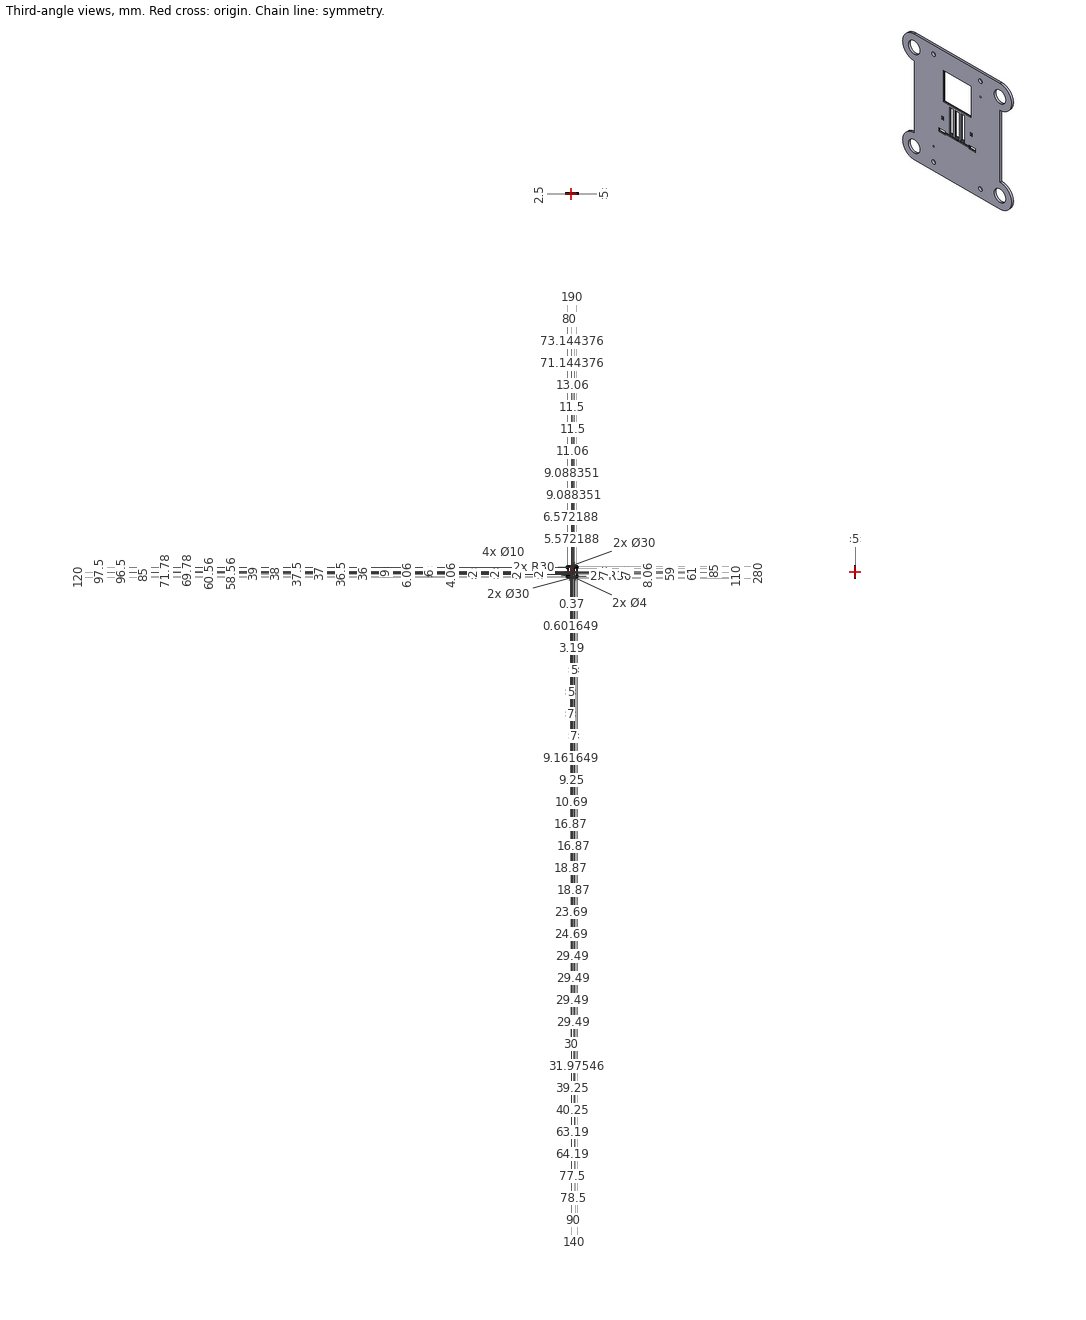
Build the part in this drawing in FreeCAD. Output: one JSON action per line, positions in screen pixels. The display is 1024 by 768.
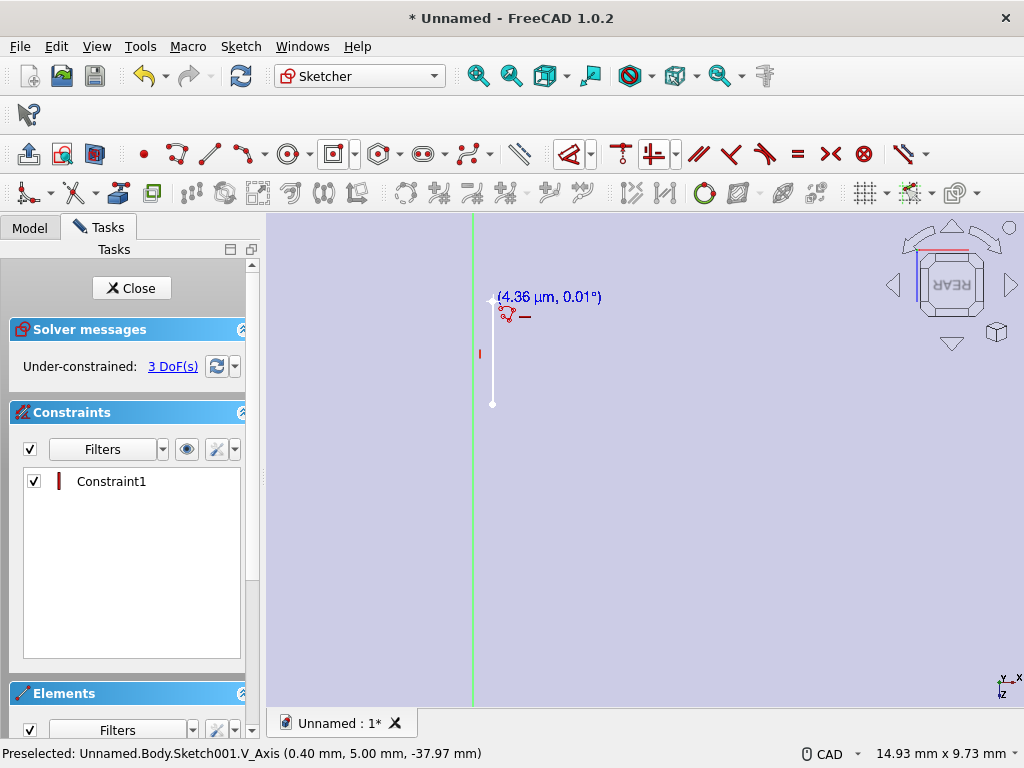
{"action": "scroll", "coordinate": [502, 299], "scroll_direction": "down", "scroll_amount": 15}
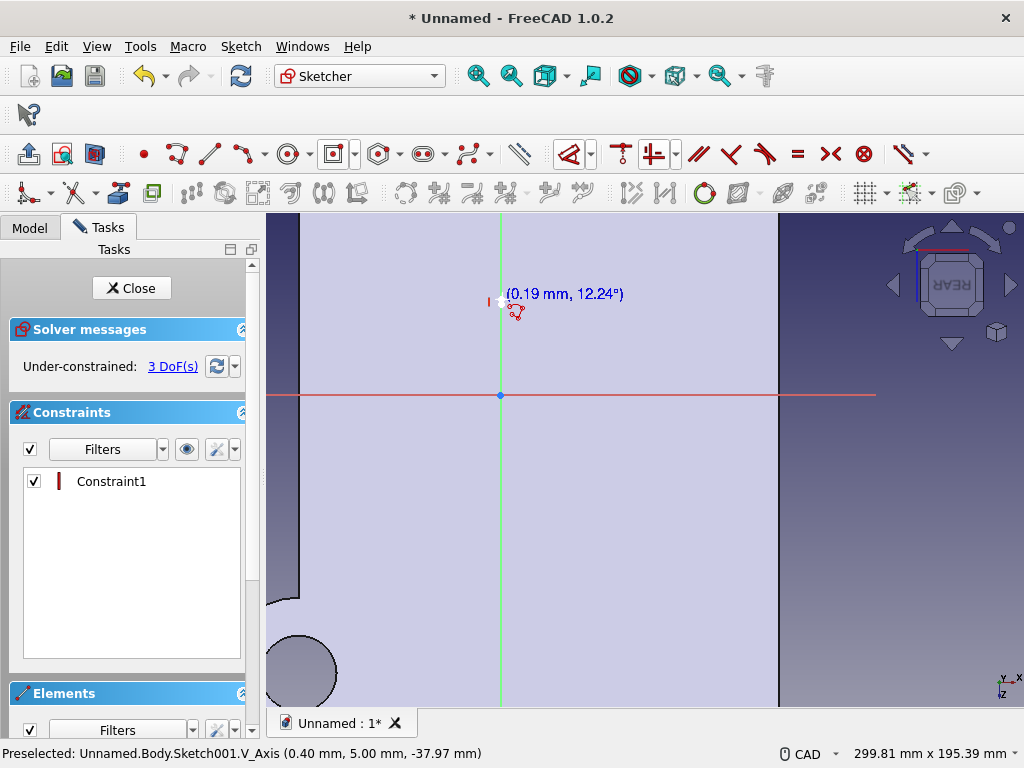
{"action": "left_click", "coordinate": [576, 299]}
{"action": "left_click", "coordinate": [576, 284]}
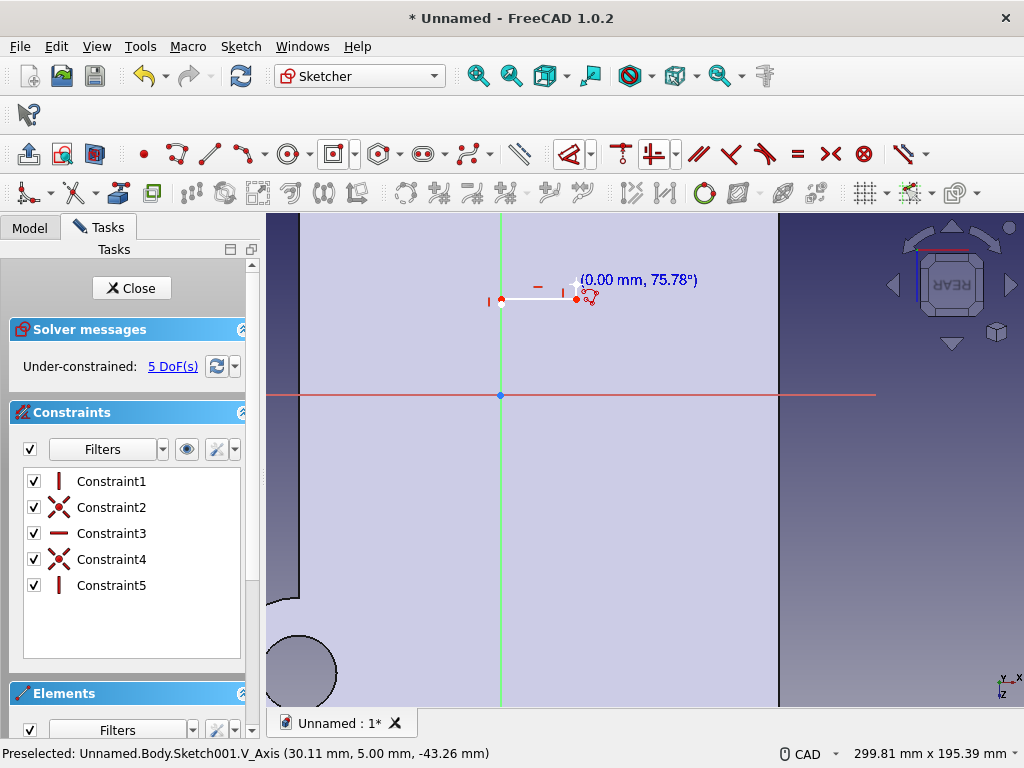
{"action": "scroll", "coordinate": [502, 284], "scroll_direction": "up", "scroll_amount": 15}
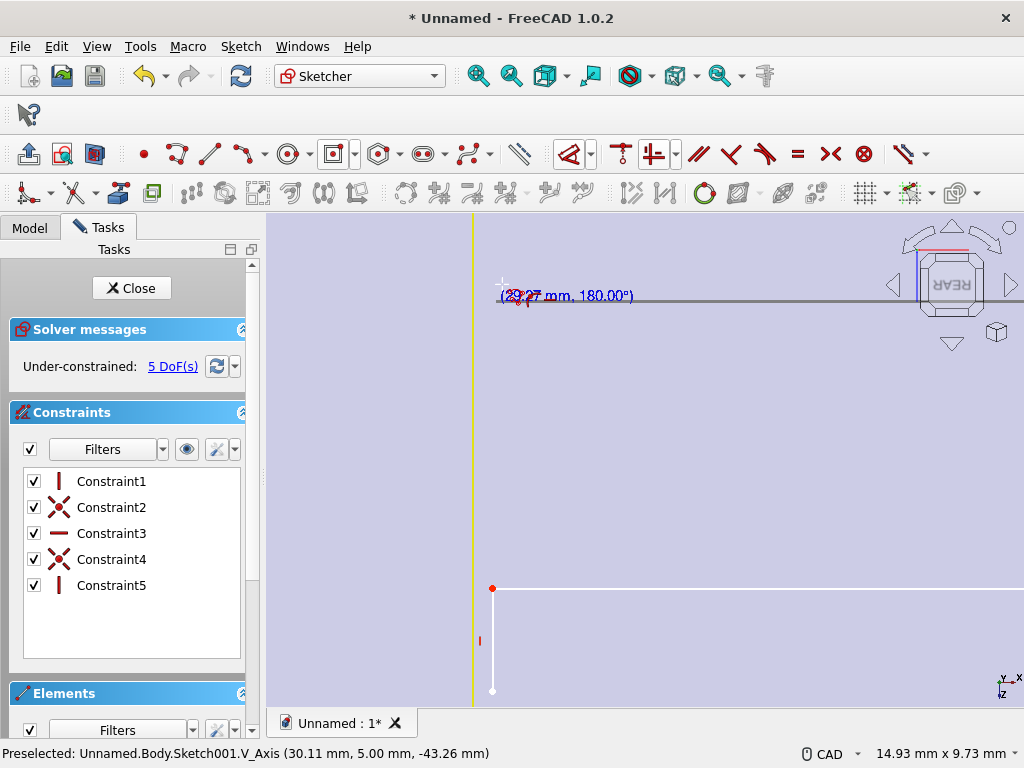
{"action": "left_click", "coordinate": [492, 281]}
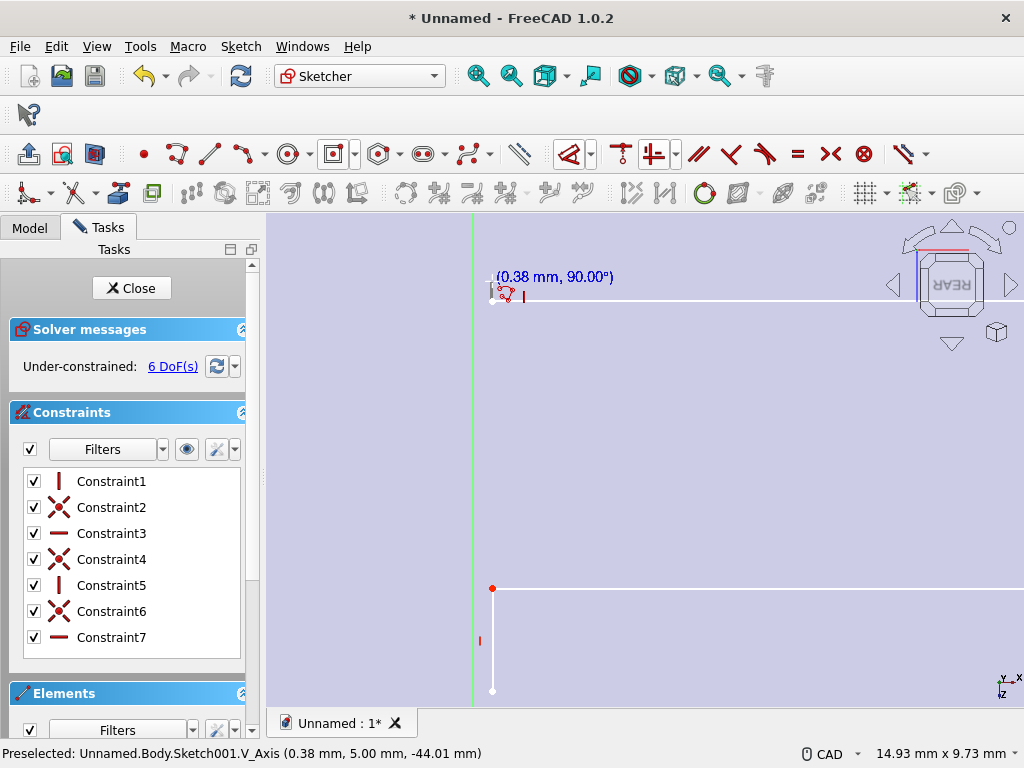
{"action": "scroll", "coordinate": [502, 284], "scroll_direction": "down", "scroll_amount": 15}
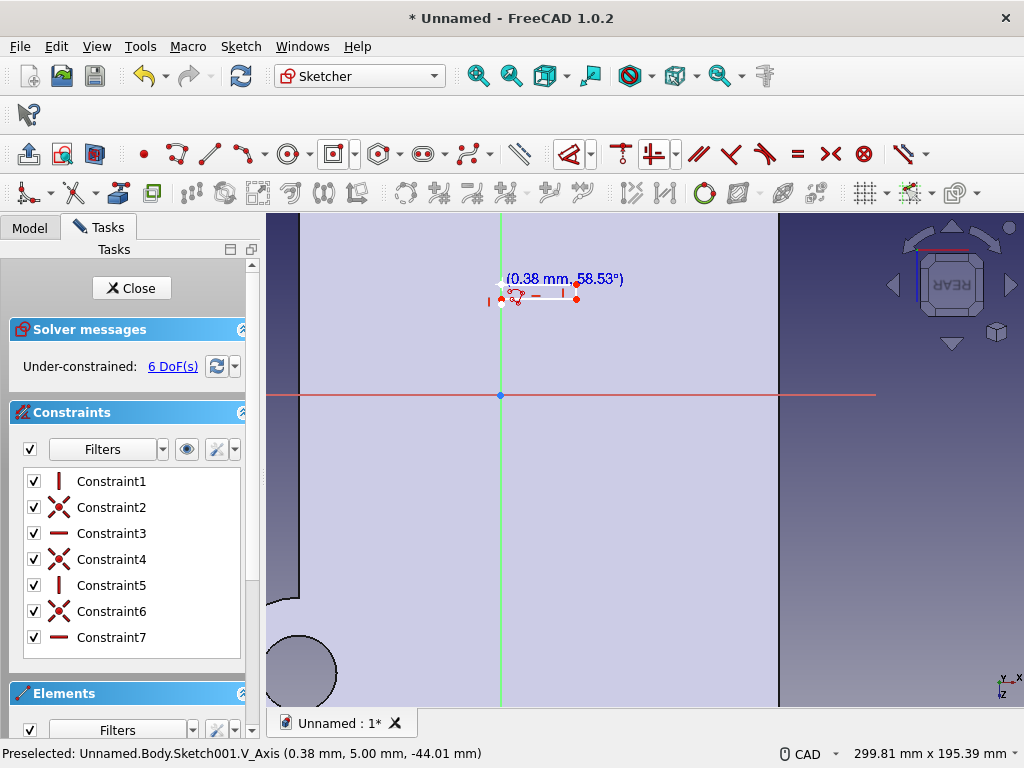
{"action": "scroll", "coordinate": [502, 279], "scroll_direction": "up", "scroll_amount": 15}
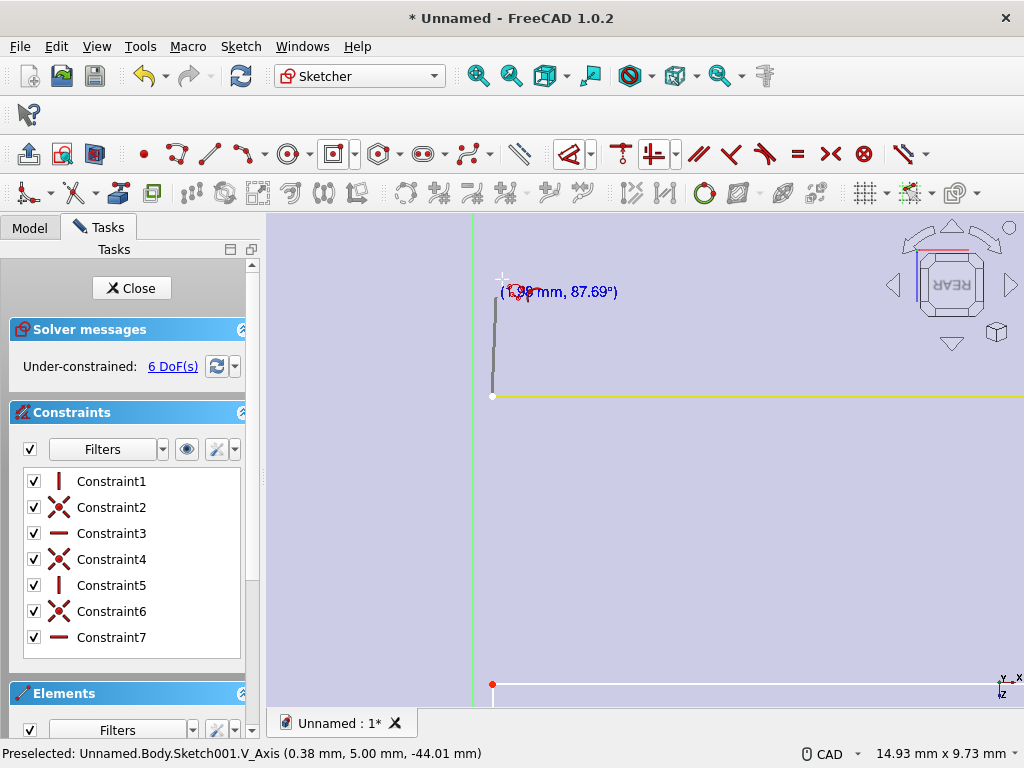
{"action": "left_click", "coordinate": [492, 275]}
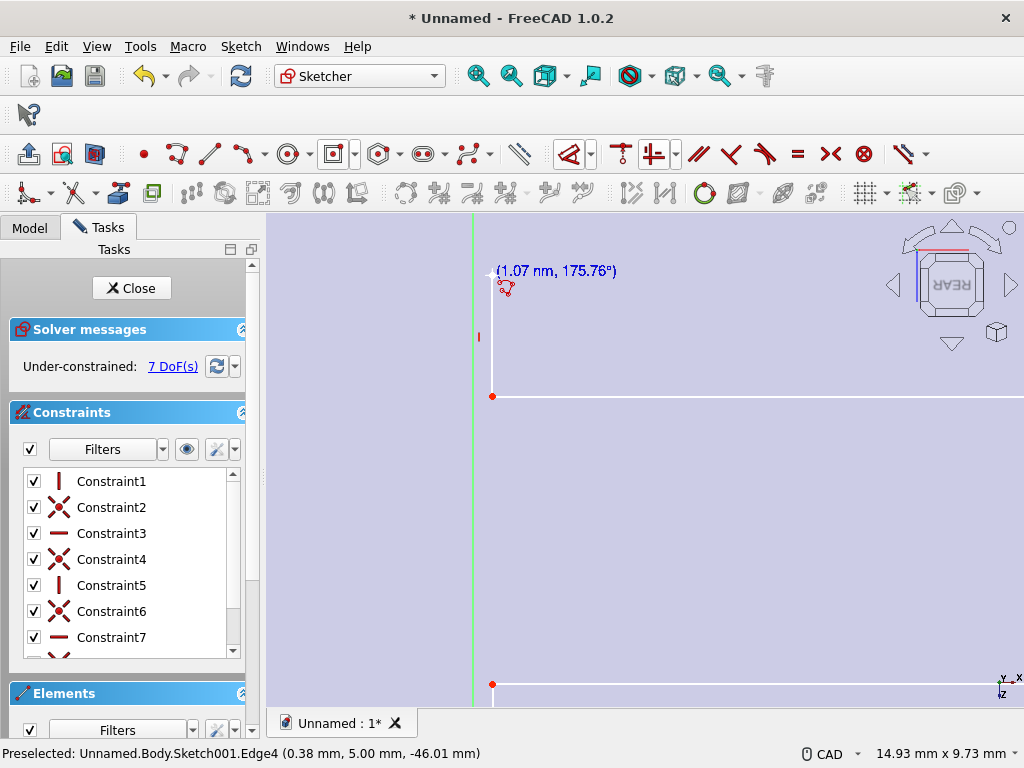
{"action": "scroll", "coordinate": [502, 279], "scroll_direction": "down", "scroll_amount": 15}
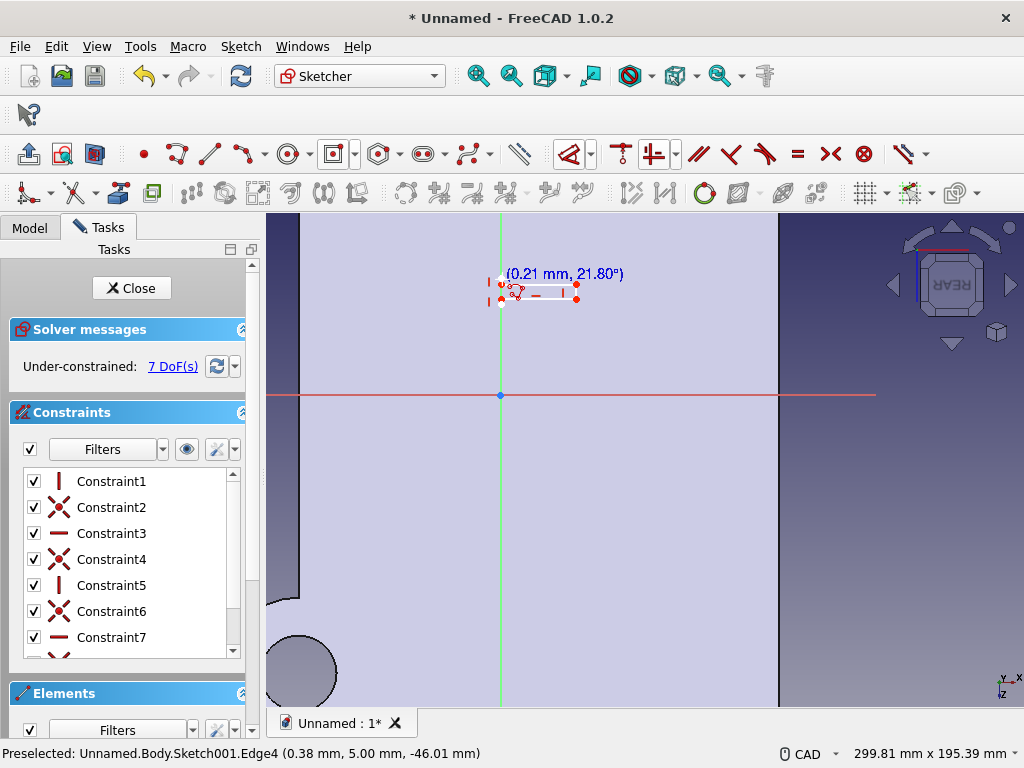
{"action": "left_click", "coordinate": [454, 279]}
{"action": "left_click", "coordinate": [454, 304]}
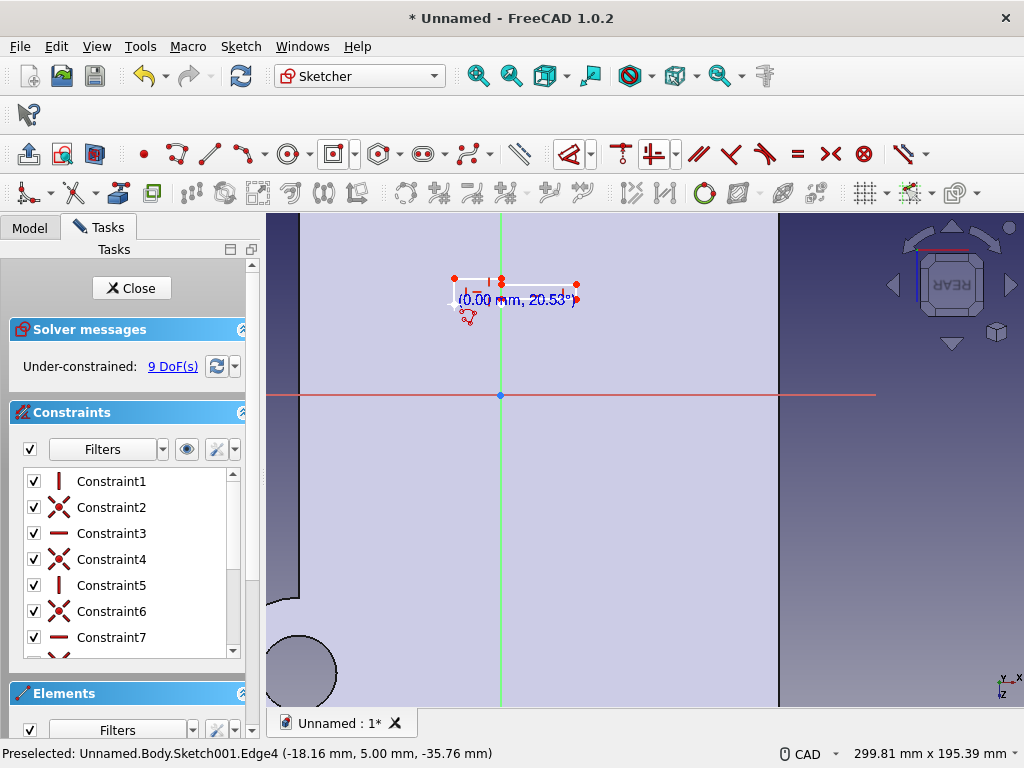
{"action": "scroll", "coordinate": [502, 304], "scroll_direction": "up", "scroll_amount": 15}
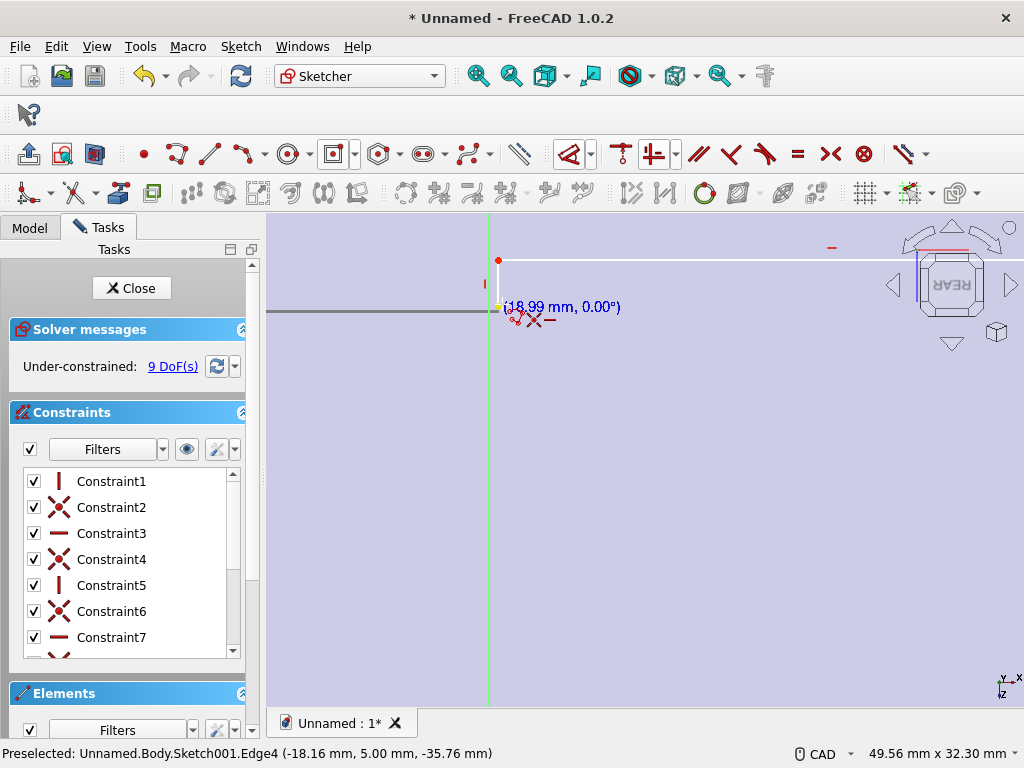
{"action": "left_click", "coordinate": [493, 309]}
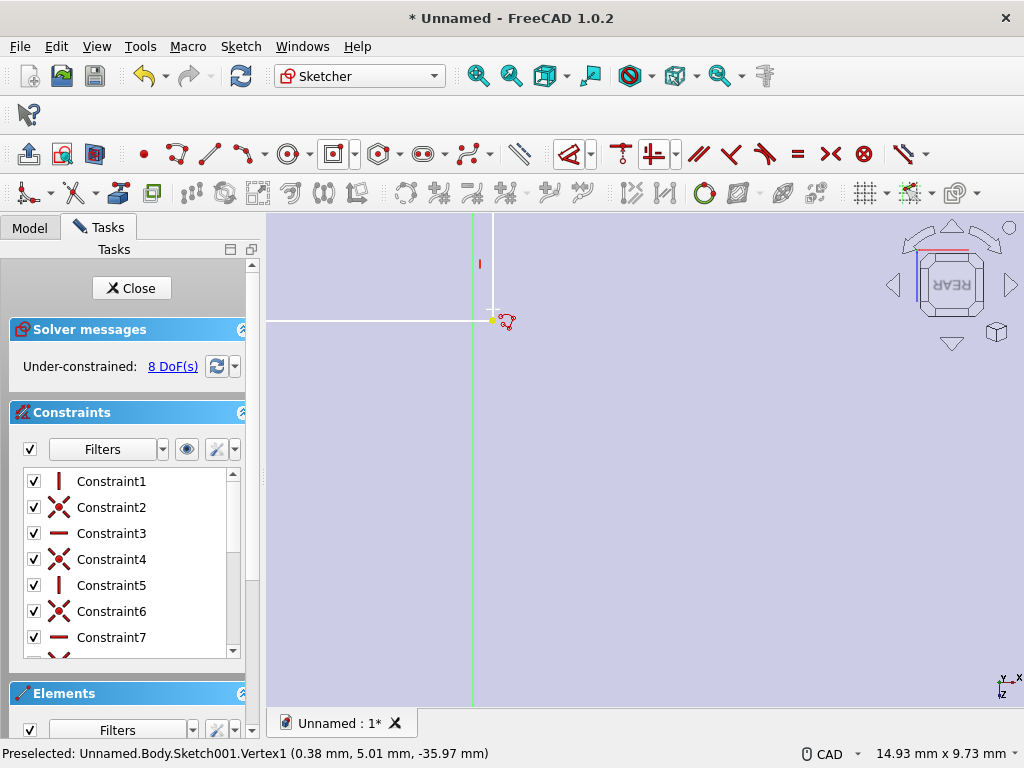
{"action": "left_click", "coordinate": [354, 154]}